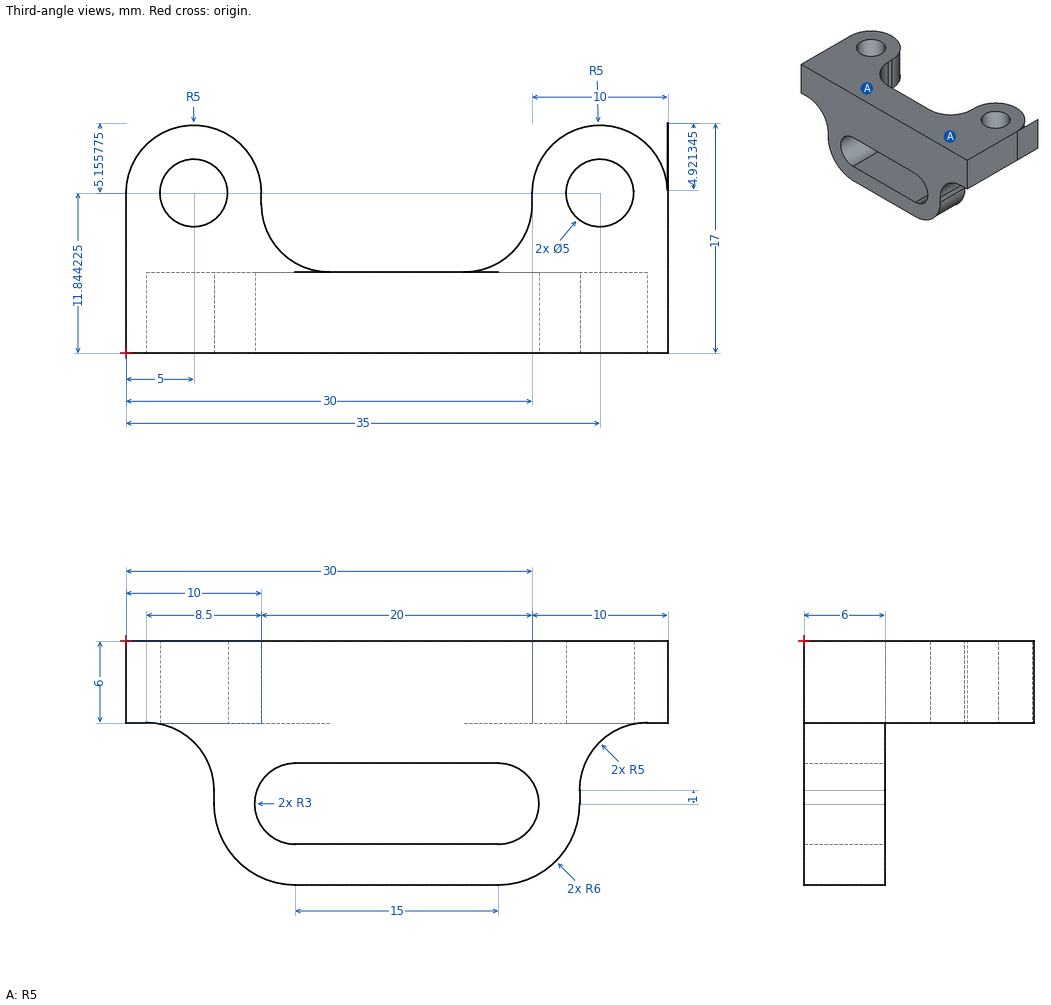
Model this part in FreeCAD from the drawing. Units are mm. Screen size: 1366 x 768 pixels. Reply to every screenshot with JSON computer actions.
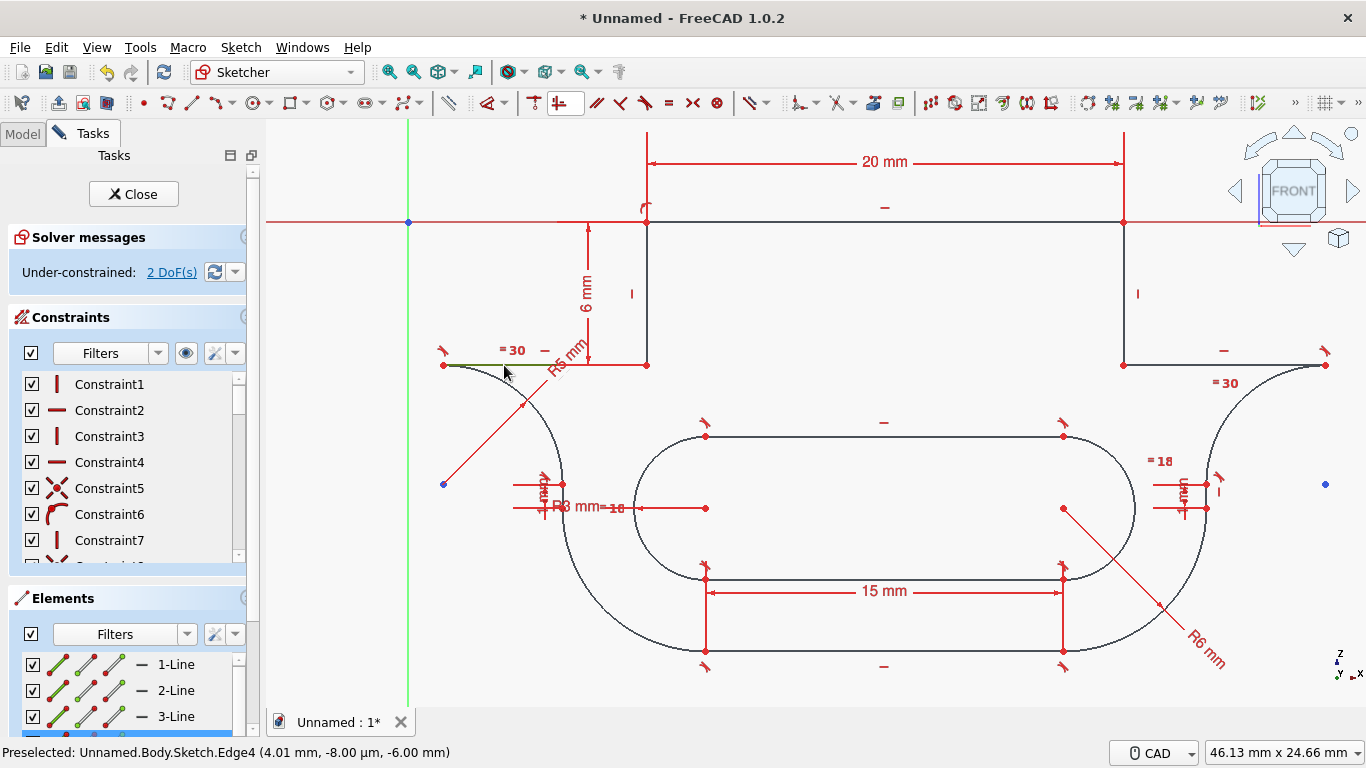
{"action": "left_click", "coordinate": [506, 104]}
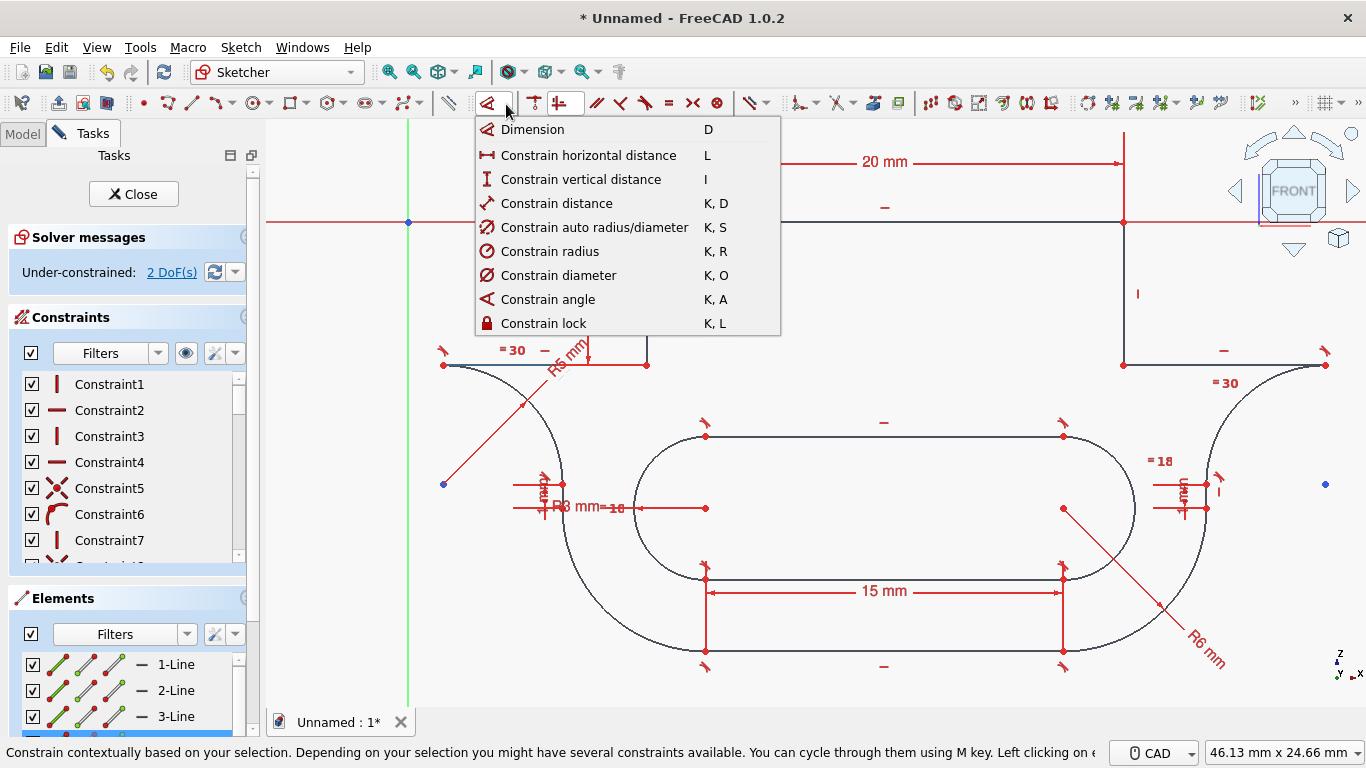
{"action": "left_click", "coordinate": [628, 155]}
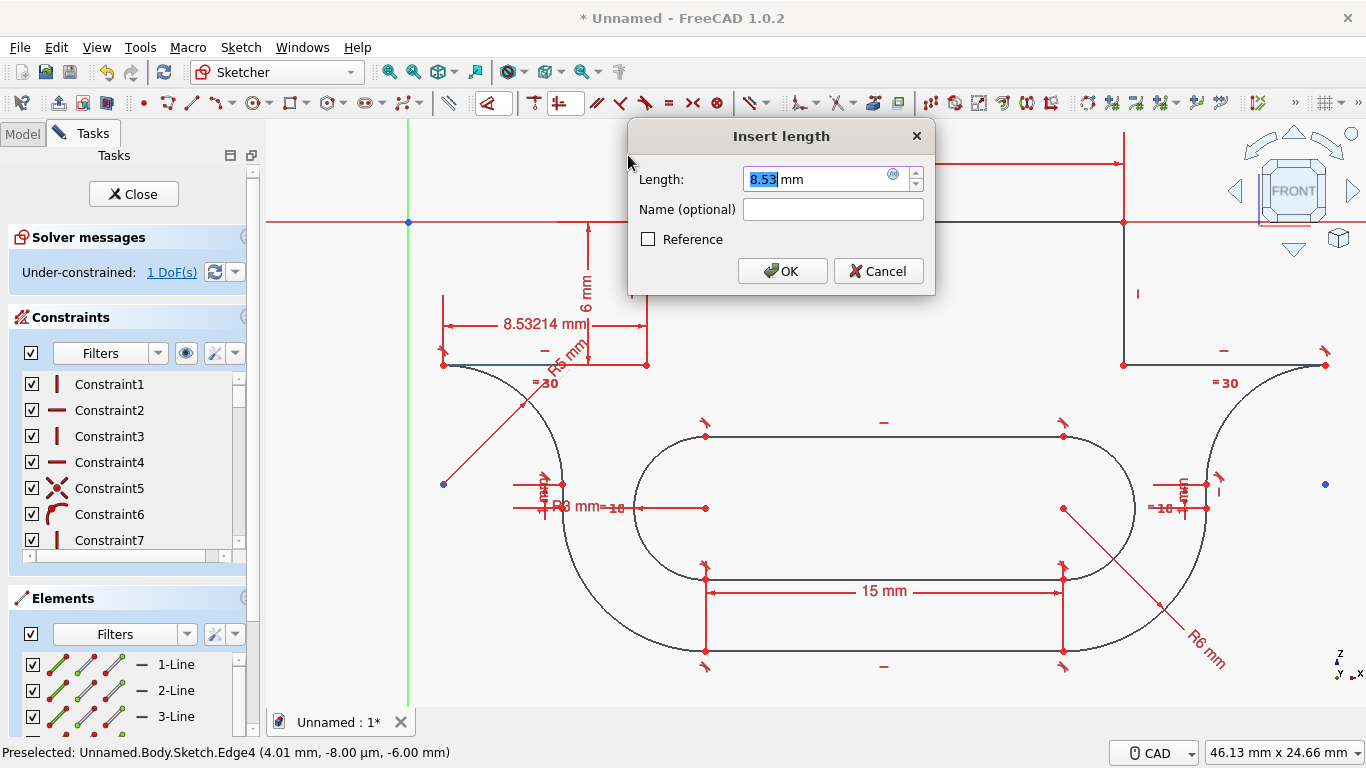
{"action": "type", "text": "8.5"}
{"action": "key", "text": "Return"}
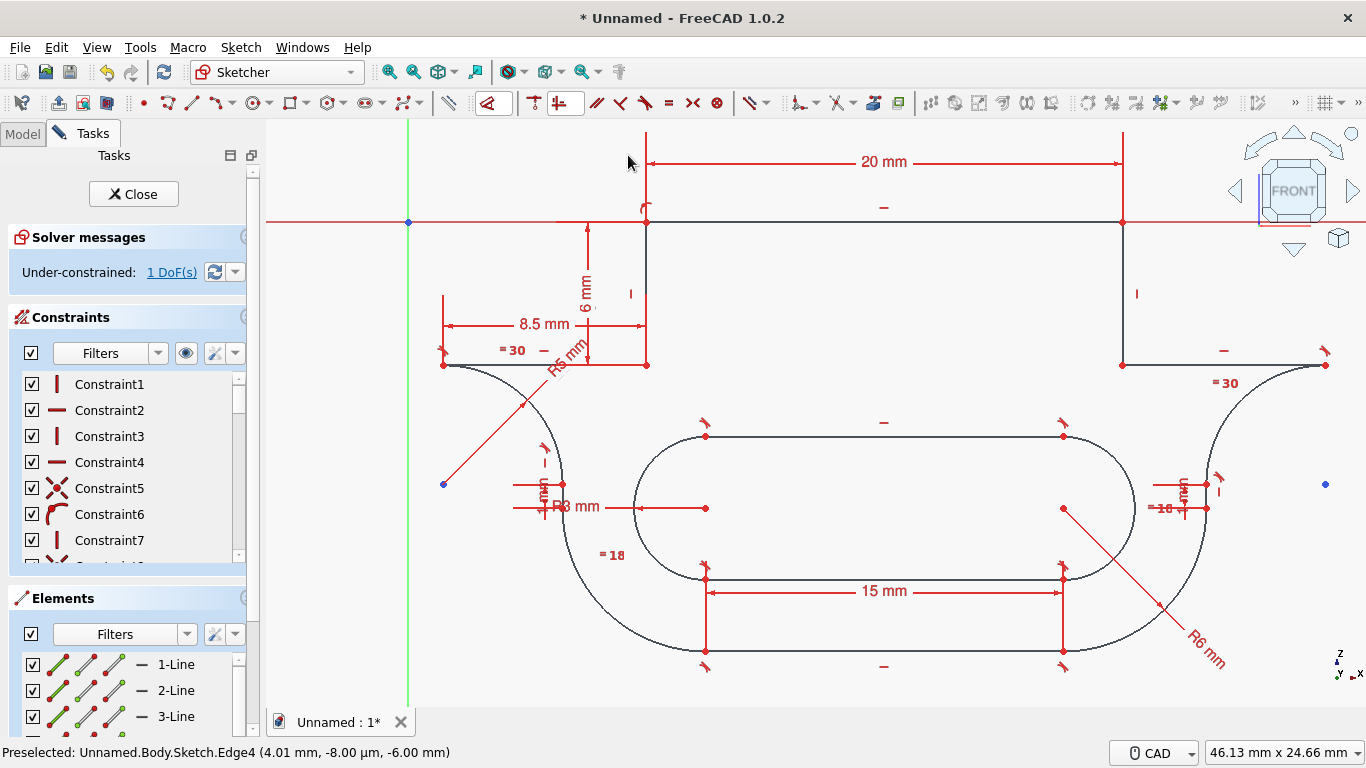
{"action": "left_click", "coordinate": [646, 365]}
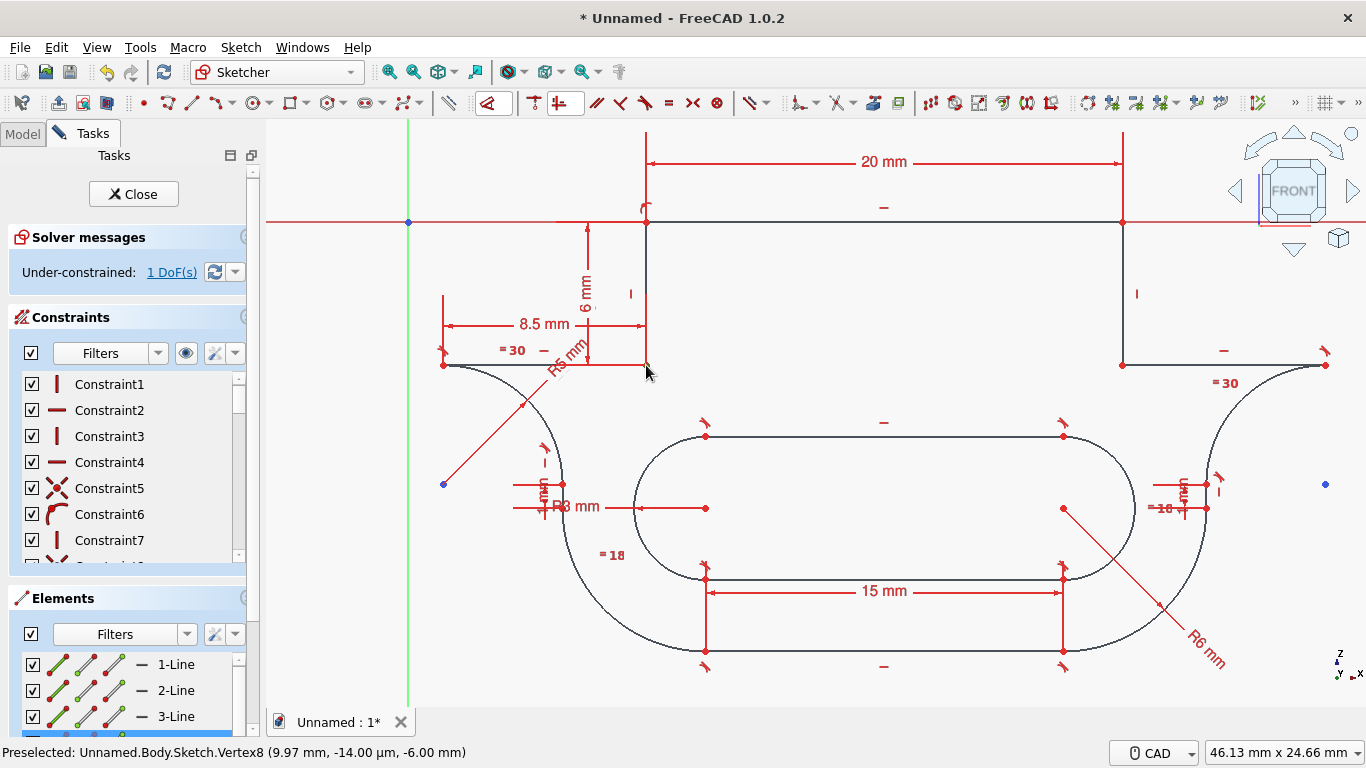
{"action": "key", "text": "l"}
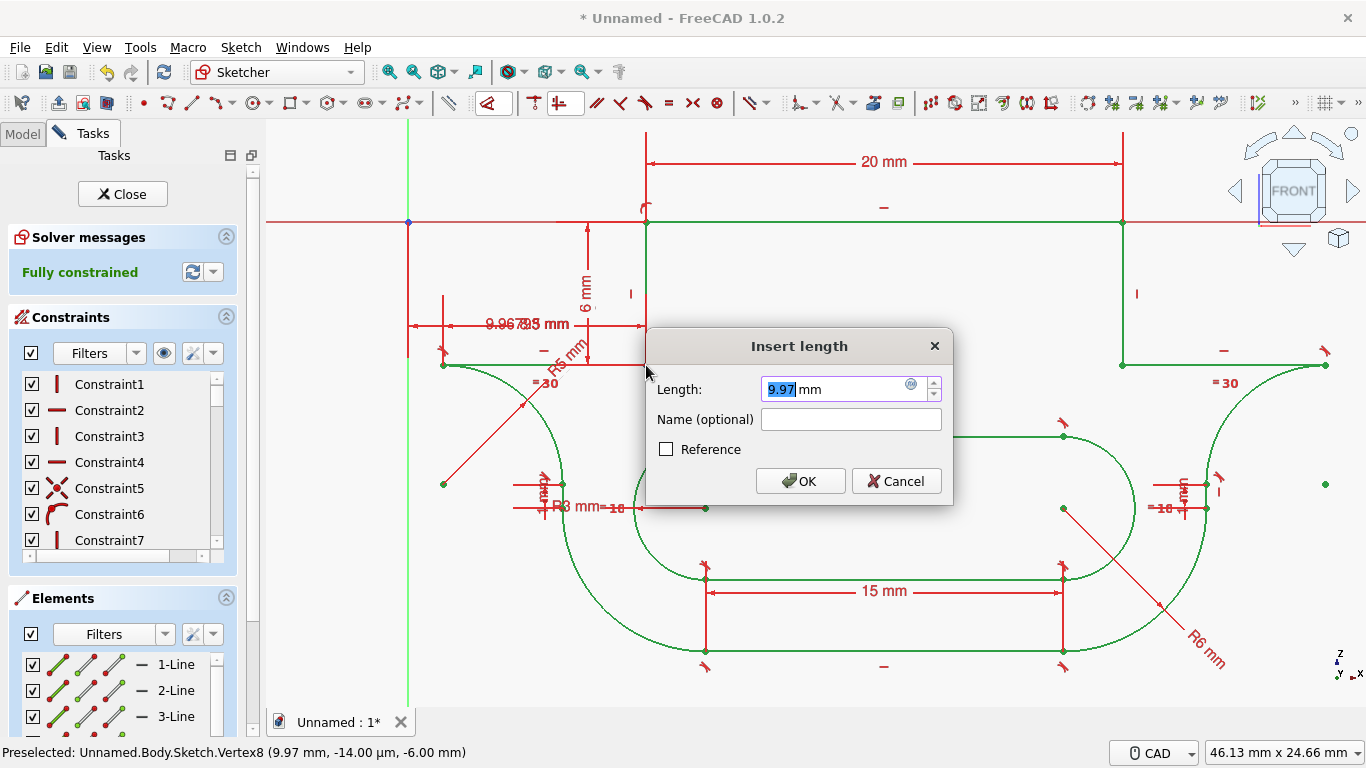
{"action": "type", "text": "10"}
{"action": "key", "text": "Return"}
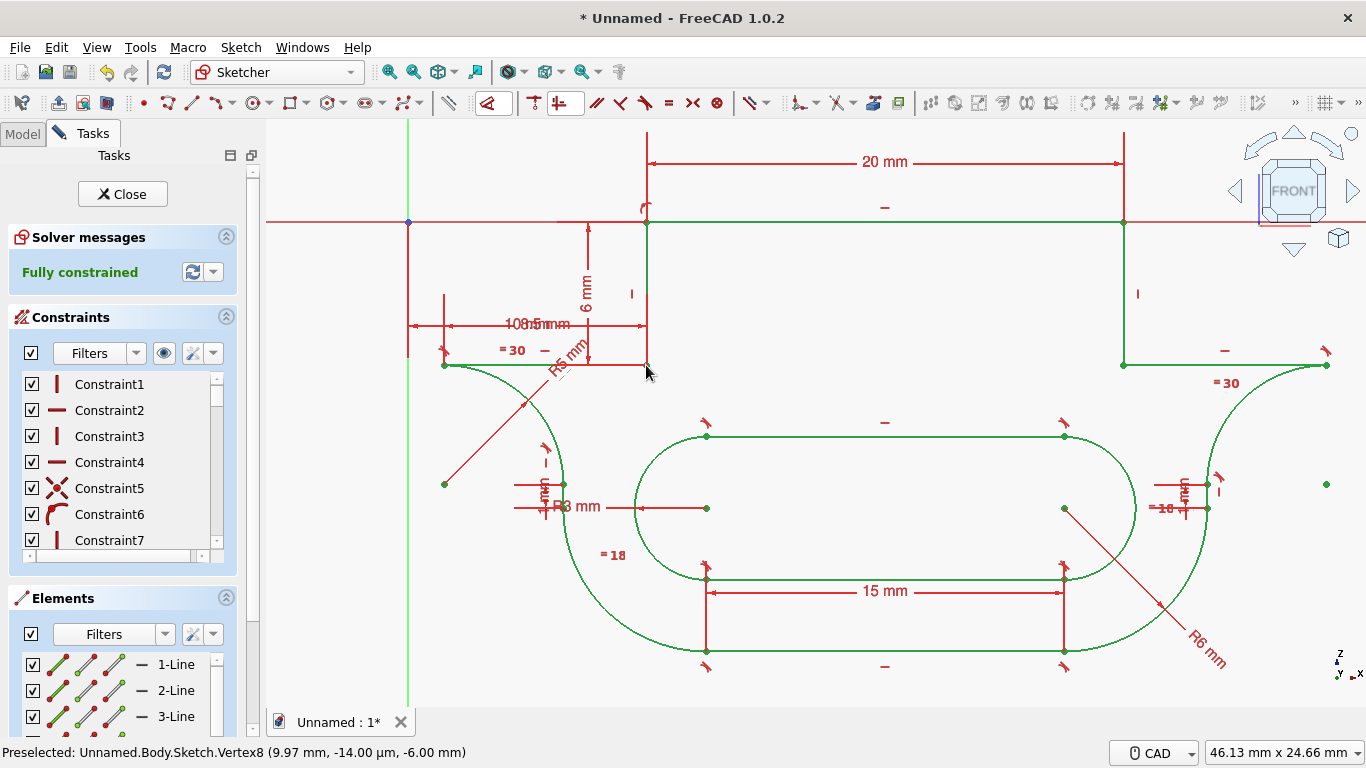
{"action": "left_click", "coordinate": [123, 194]}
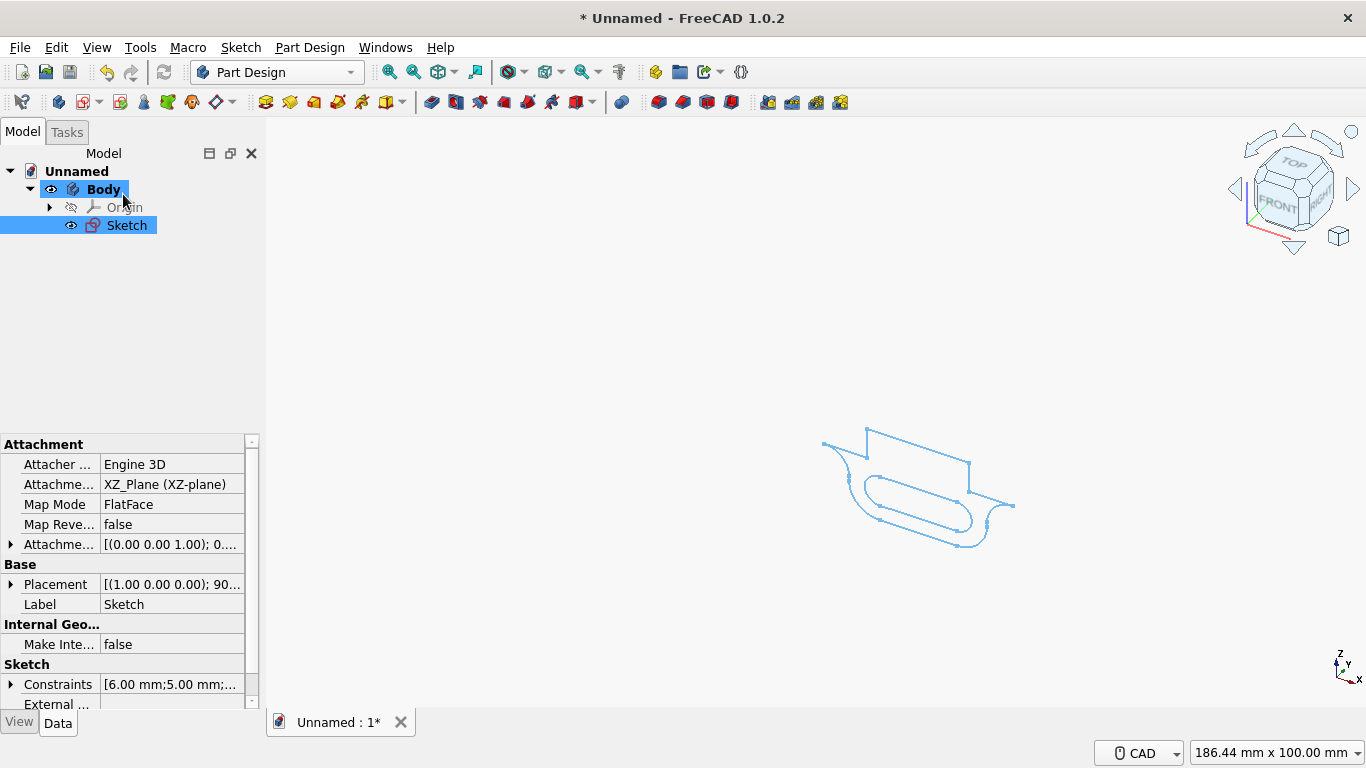
{"action": "left_click", "coordinate": [266, 102]}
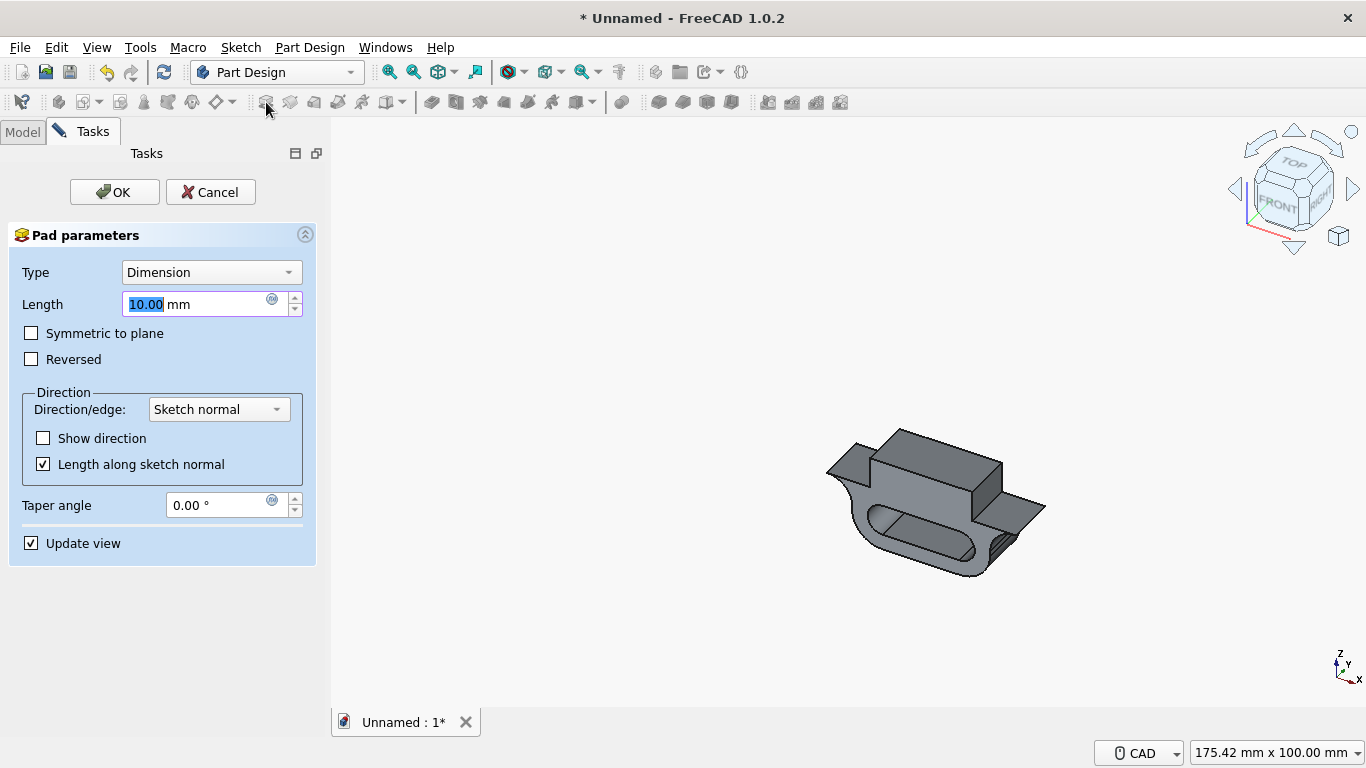
{"action": "type", "text": "6"}
{"action": "key", "text": "Tab"}